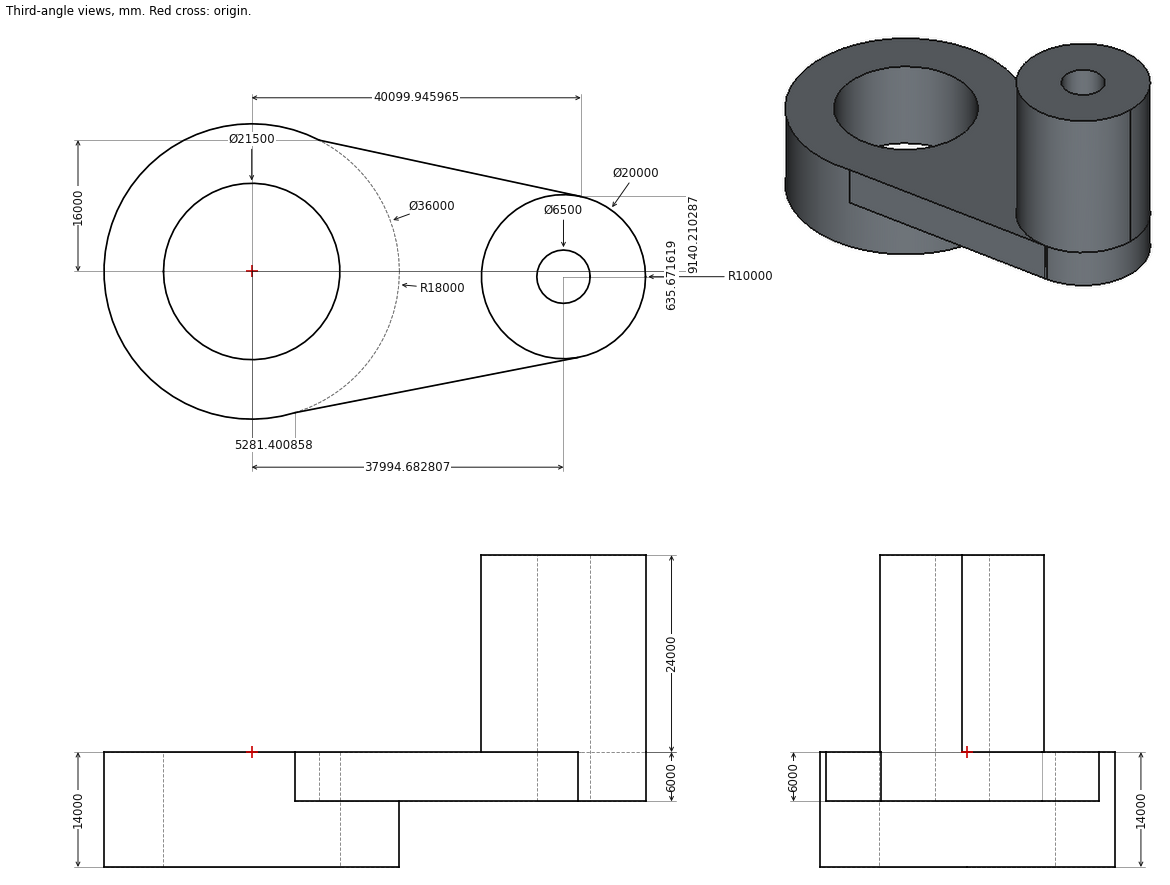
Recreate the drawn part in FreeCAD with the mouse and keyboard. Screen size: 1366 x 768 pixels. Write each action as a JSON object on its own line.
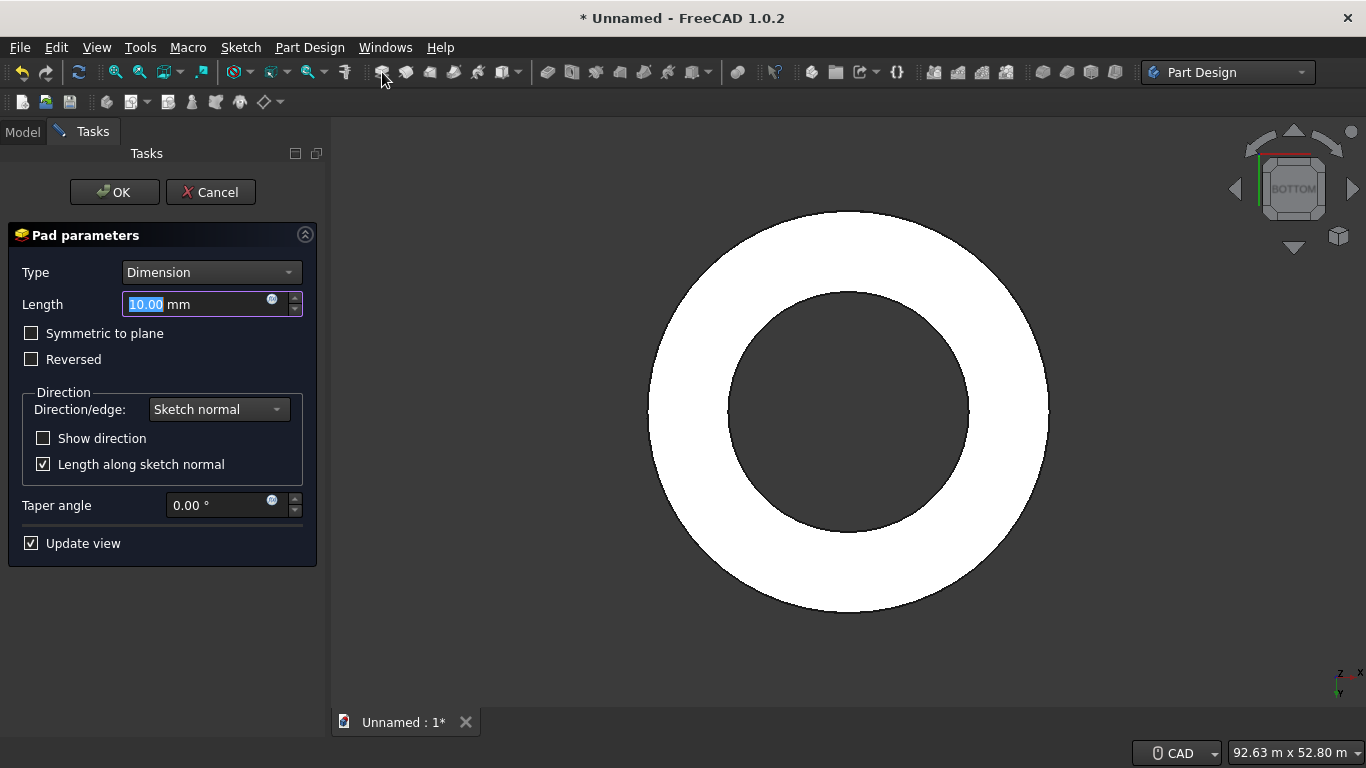
{"action": "type", "text": "6000"}
{"action": "key", "text": "Tab"}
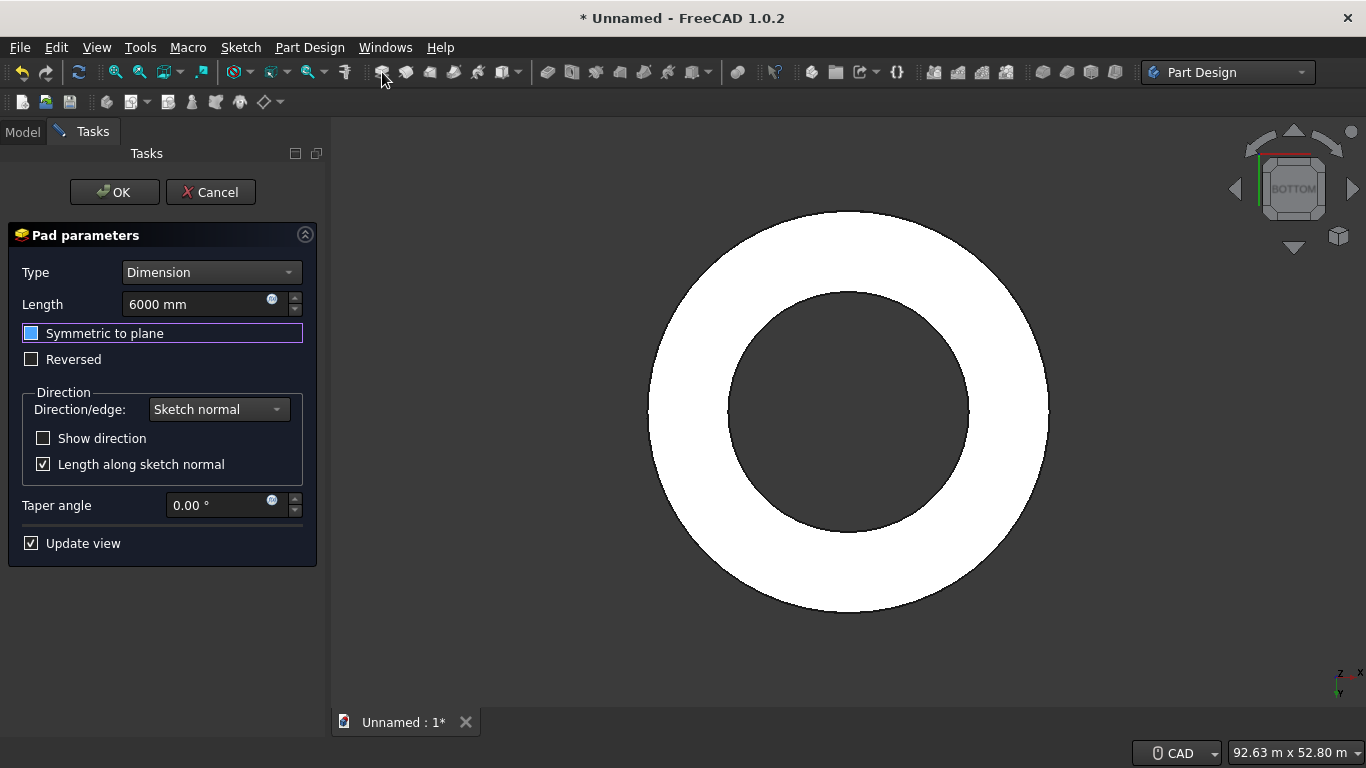
{"action": "left_click", "coordinate": [30, 359]}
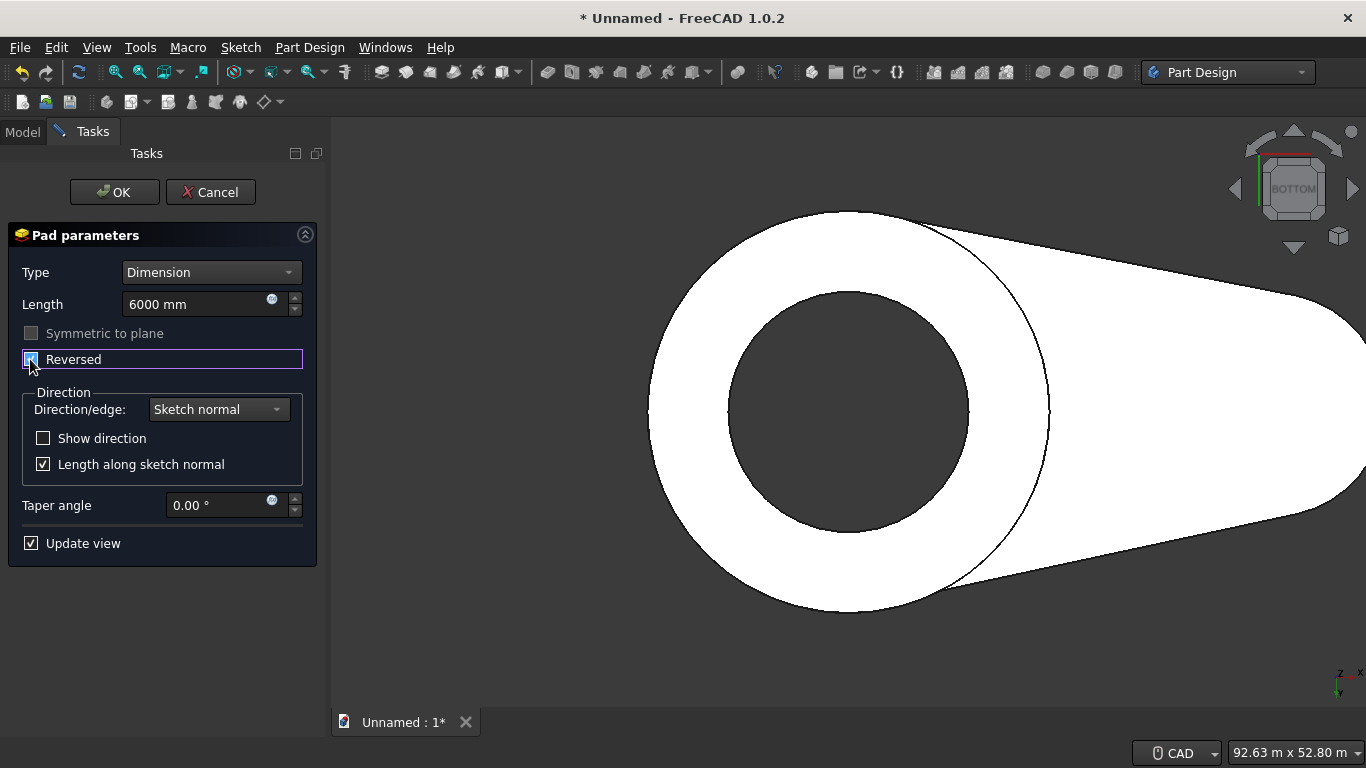
{"action": "left_click", "coordinate": [115, 192]}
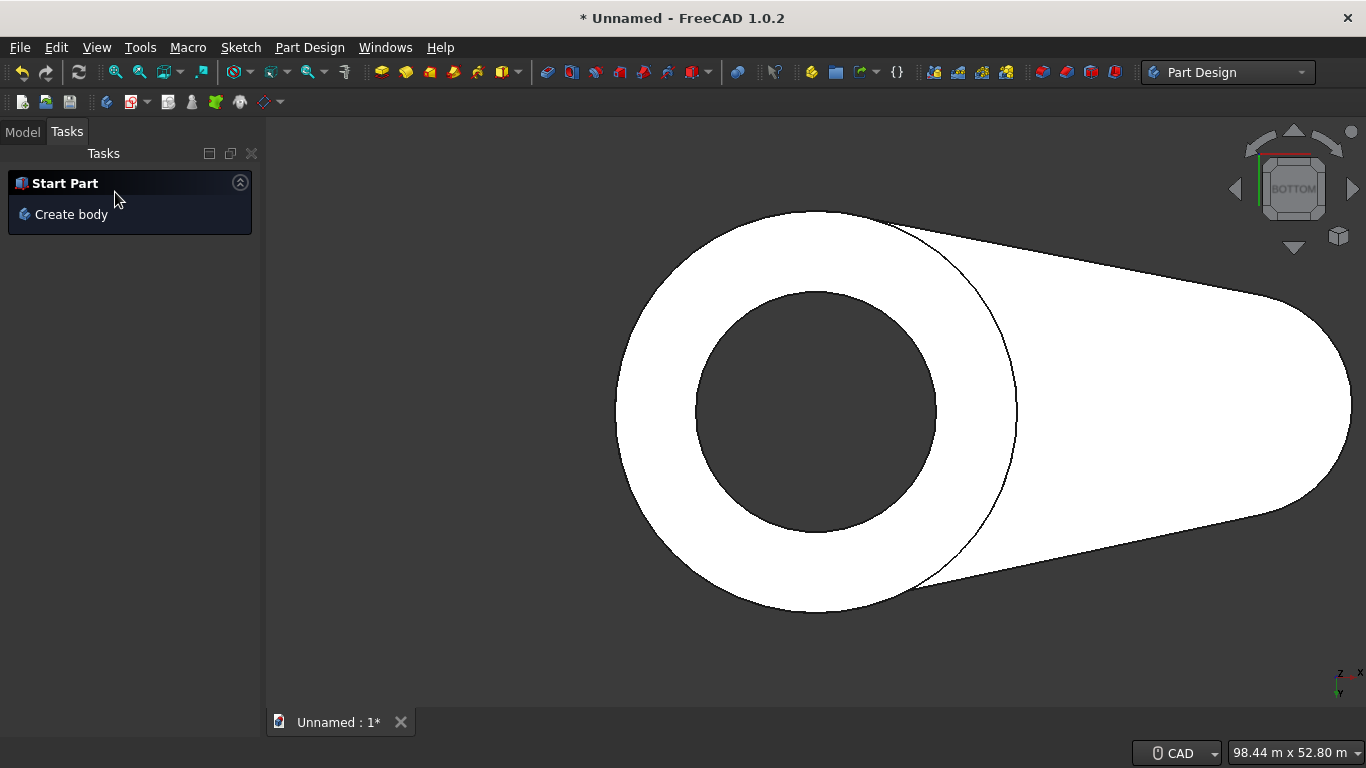
{"action": "left_click", "coordinate": [132, 102]}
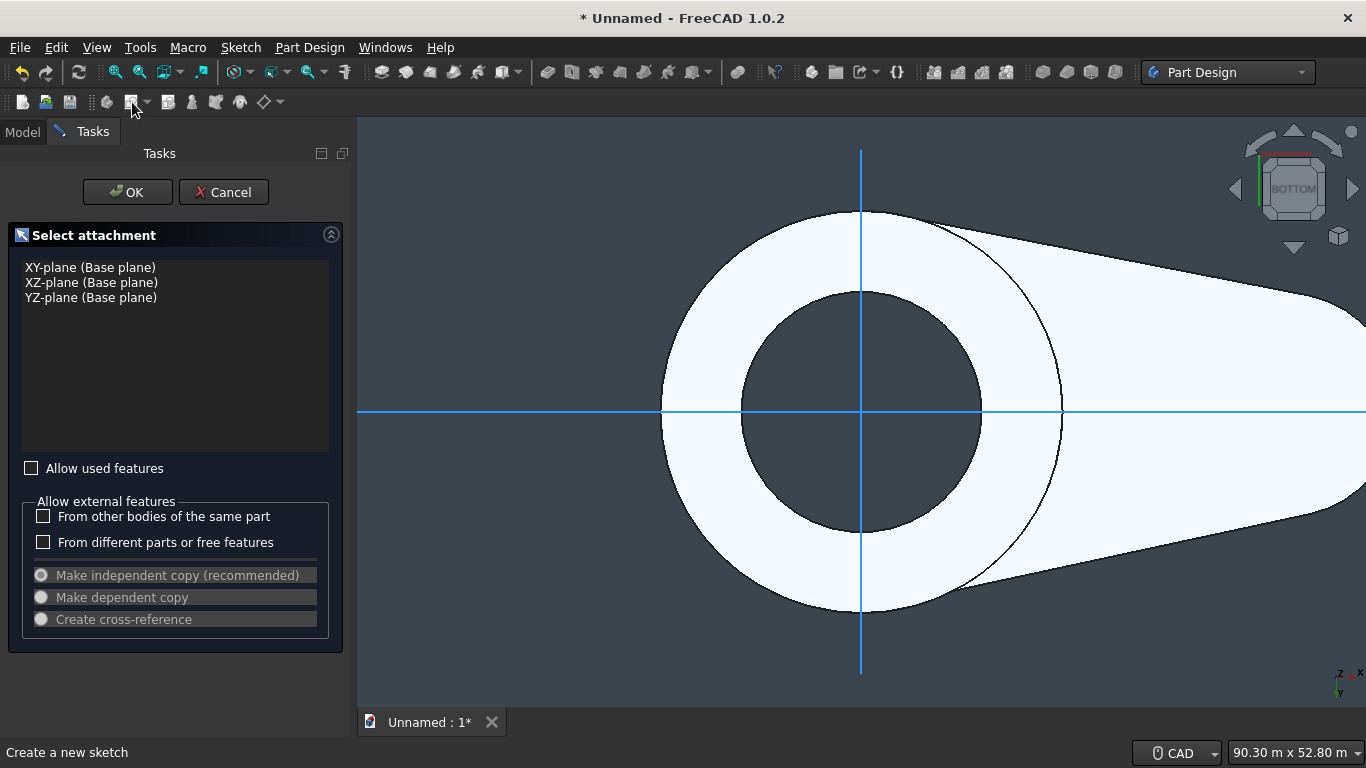
{"action": "left_click", "coordinate": [82, 268]}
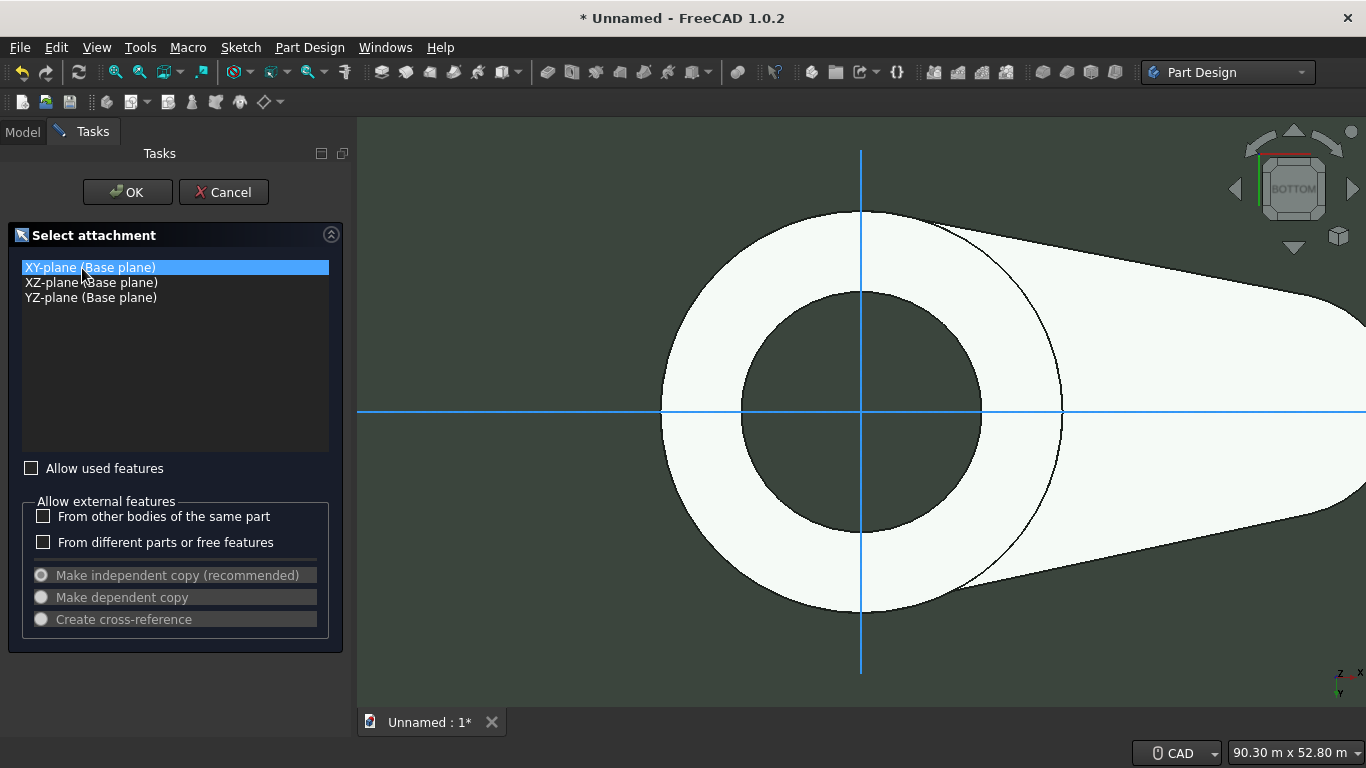
{"action": "left_click", "coordinate": [128, 192]}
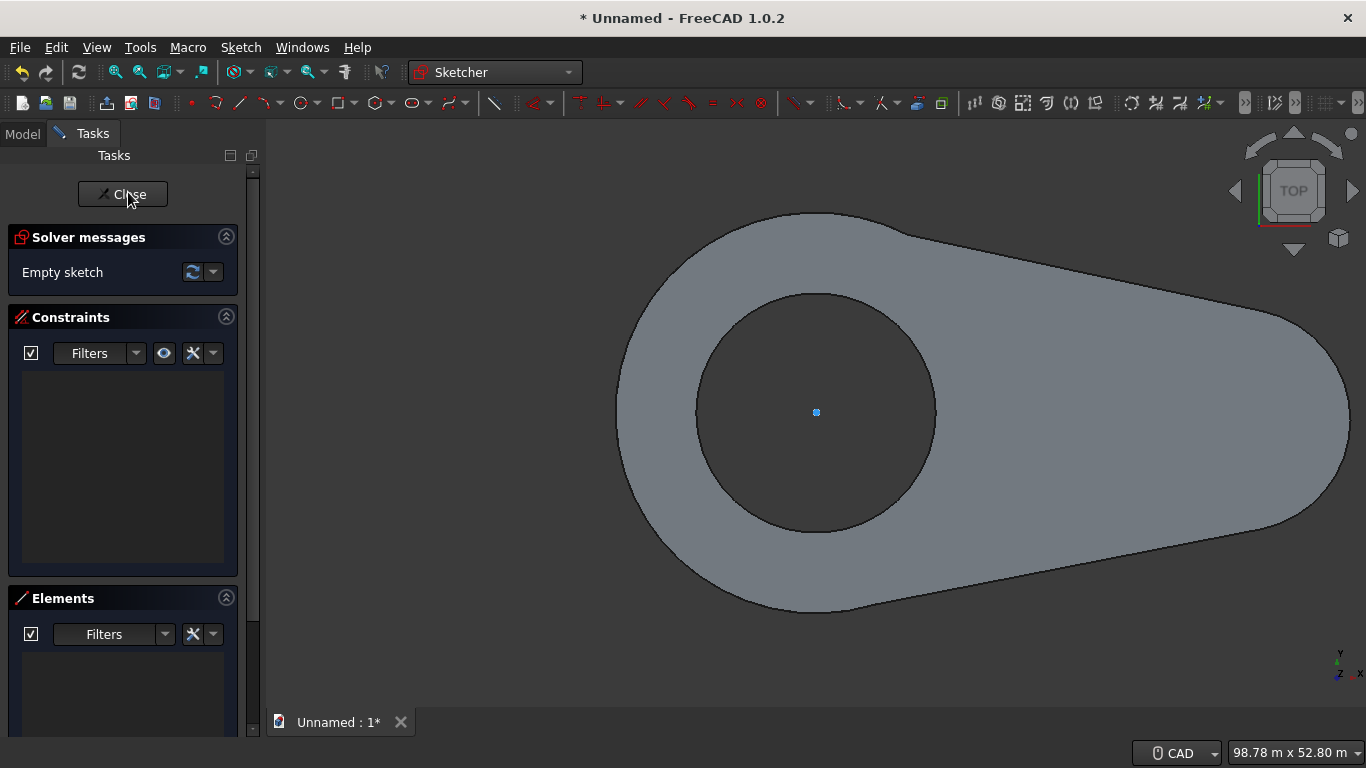
{"action": "scroll", "coordinate": [294, 381], "scroll_direction": "down", "scroll_amount": 1}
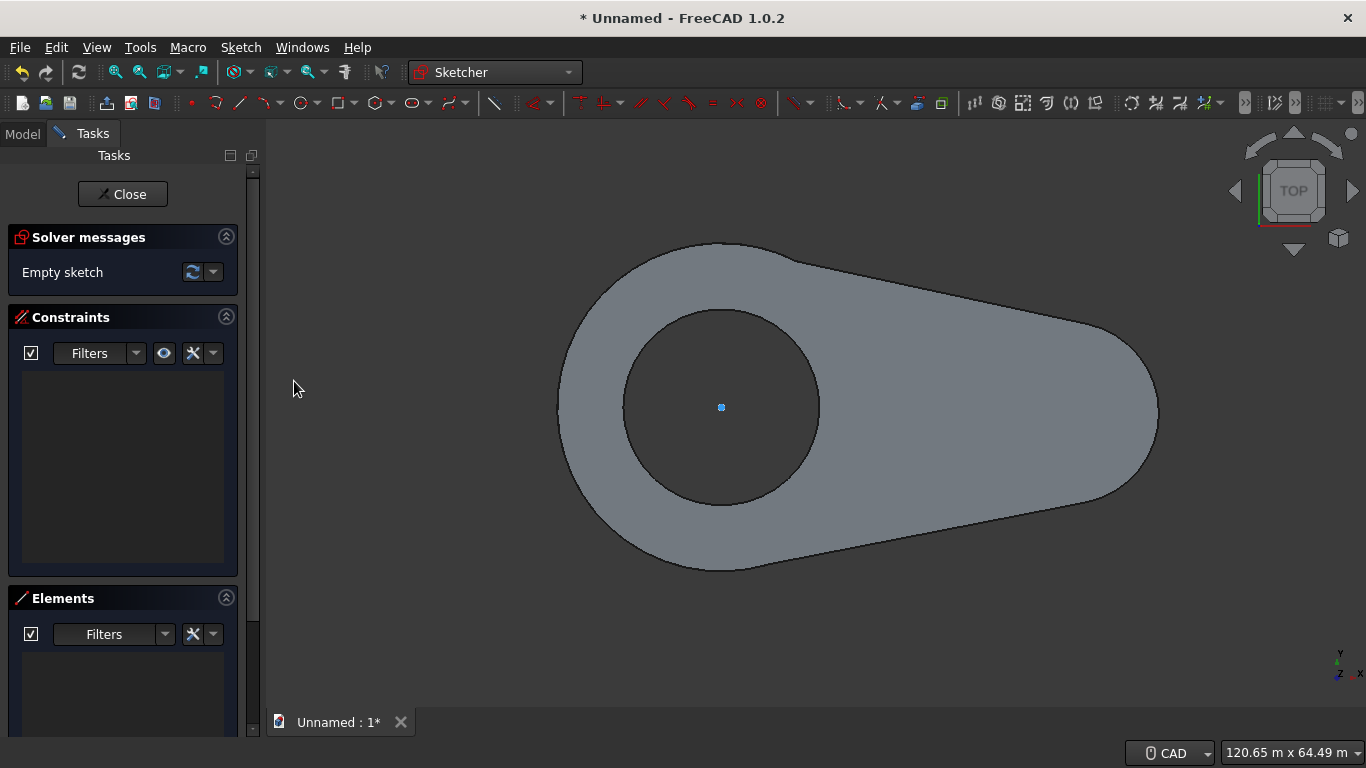
{"action": "scroll", "coordinate": [1201, 413], "scroll_direction": "up", "scroll_amount": 2}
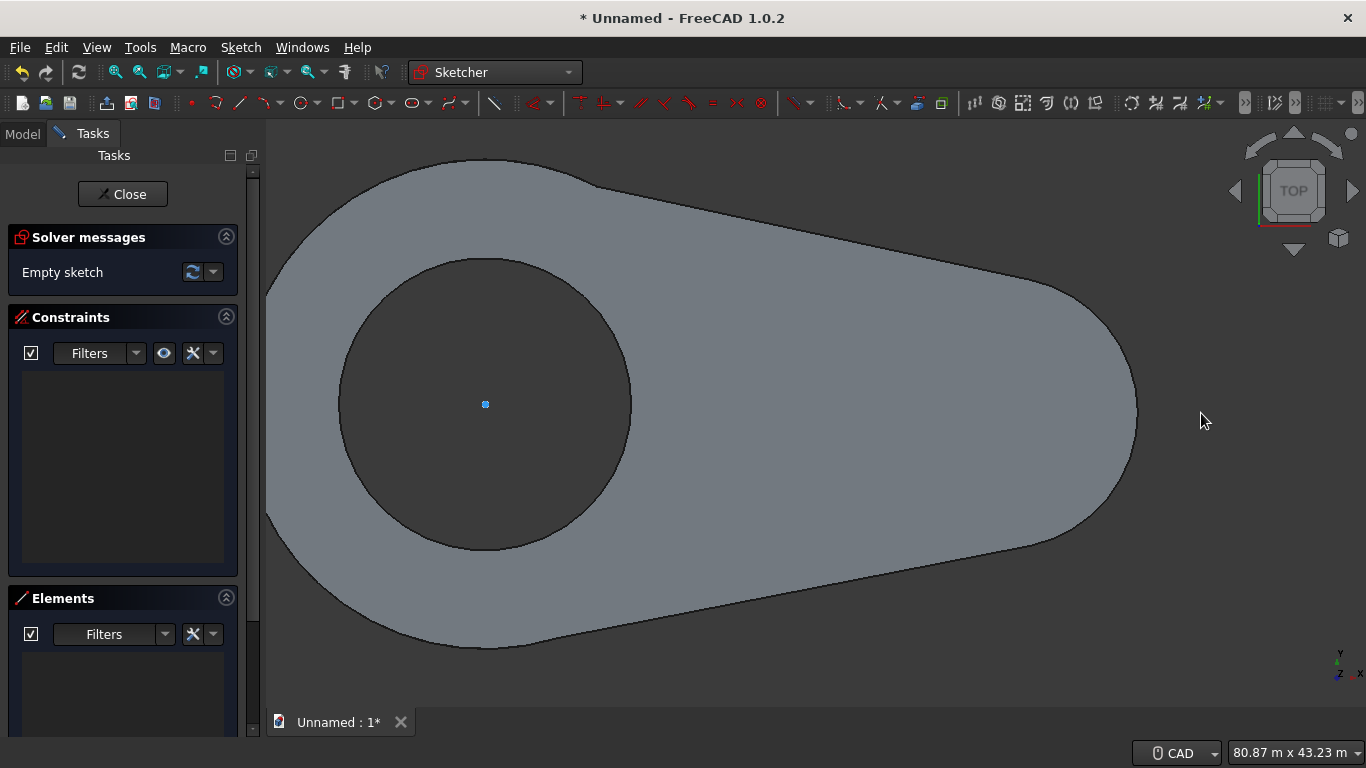
{"action": "left_click", "coordinate": [302, 104]}